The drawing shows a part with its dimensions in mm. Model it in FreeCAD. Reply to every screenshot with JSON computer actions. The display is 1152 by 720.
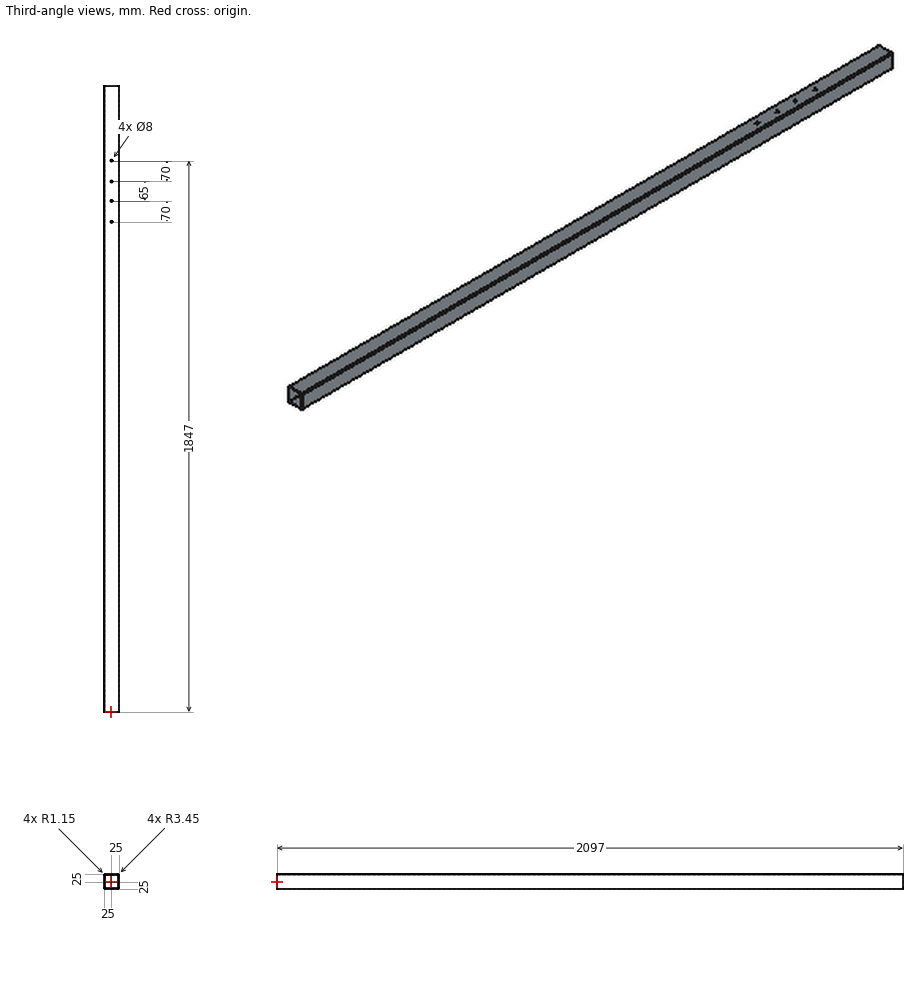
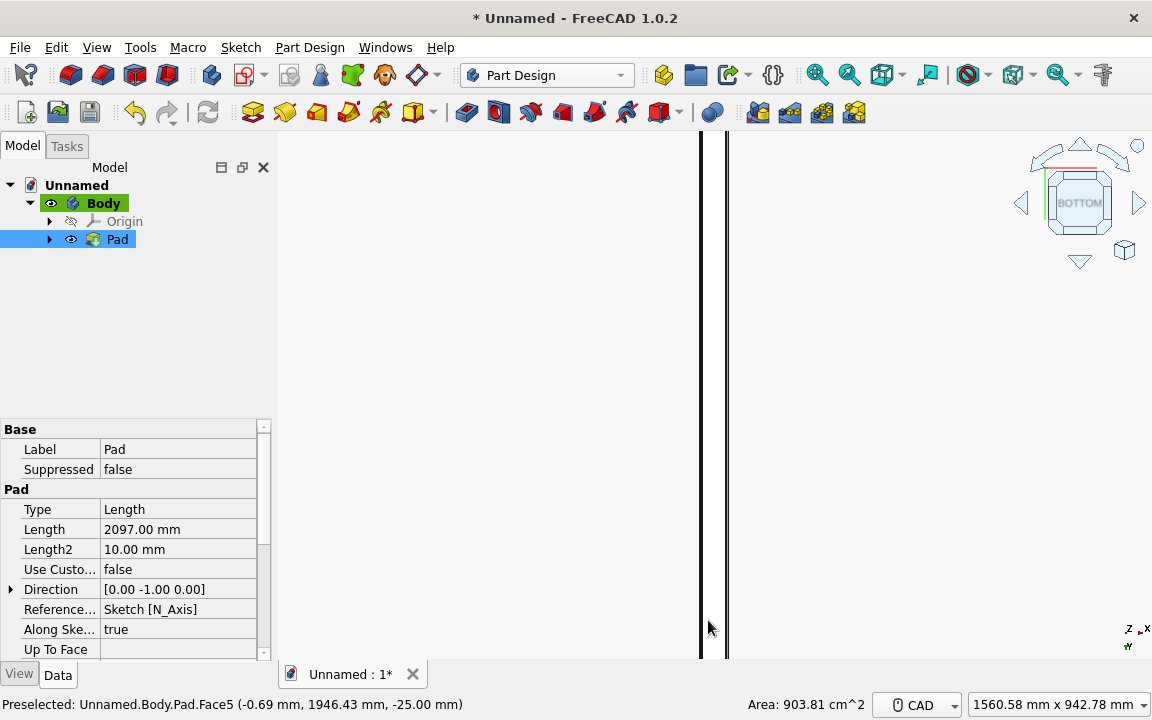
{"action": "left_click", "coordinate": [244, 76]}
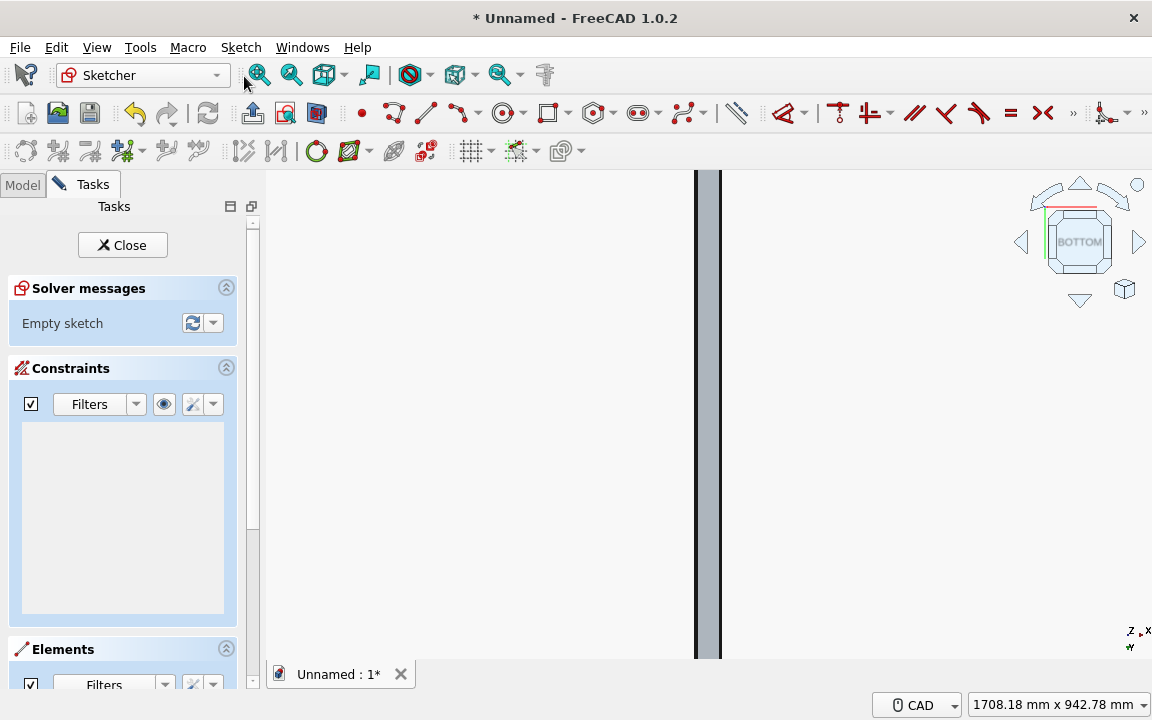
{"action": "scroll", "coordinate": [748, 580], "scroll_direction": "up", "scroll_amount": 5}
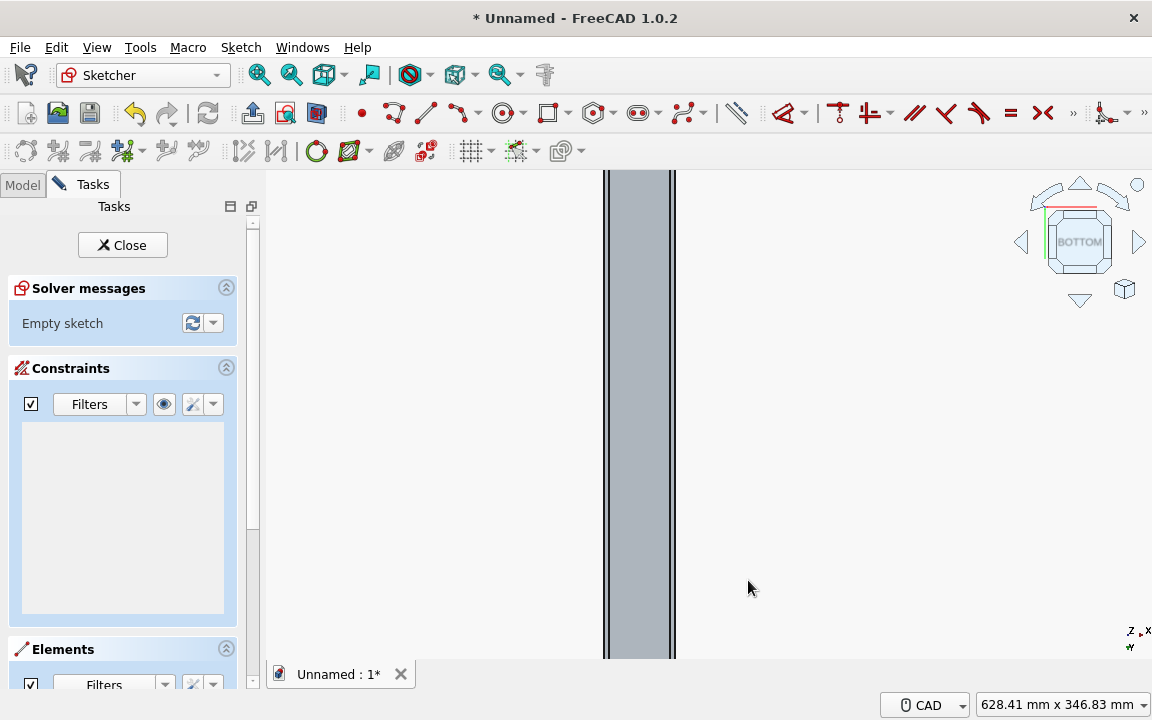
{"action": "left_click", "coordinate": [504, 114]}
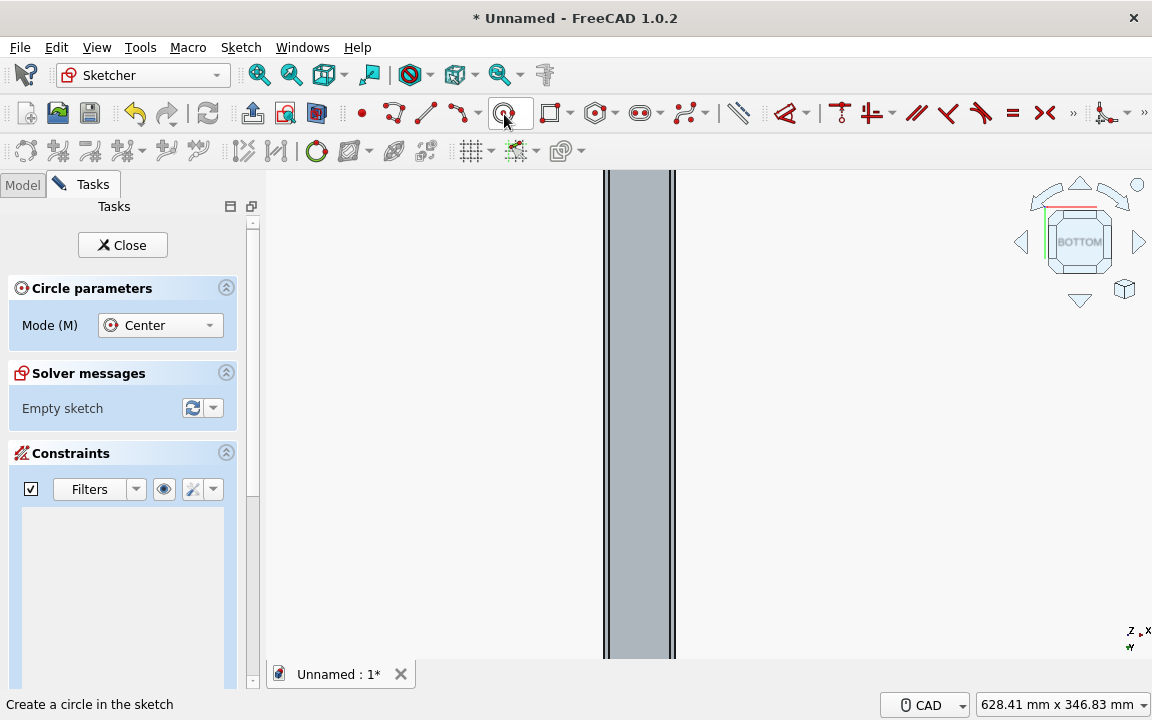
{"action": "scroll", "coordinate": [640, 557], "scroll_direction": "up", "scroll_amount": 7}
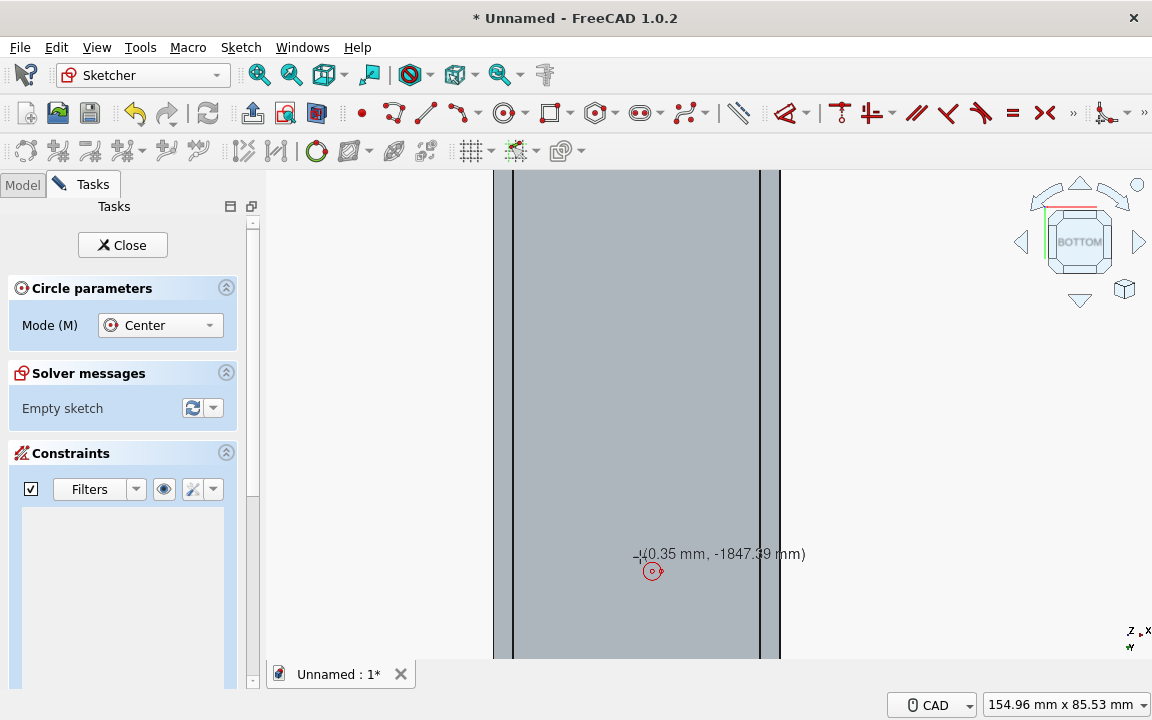
{"action": "scroll", "coordinate": [642, 560], "scroll_direction": "down", "scroll_amount": 7}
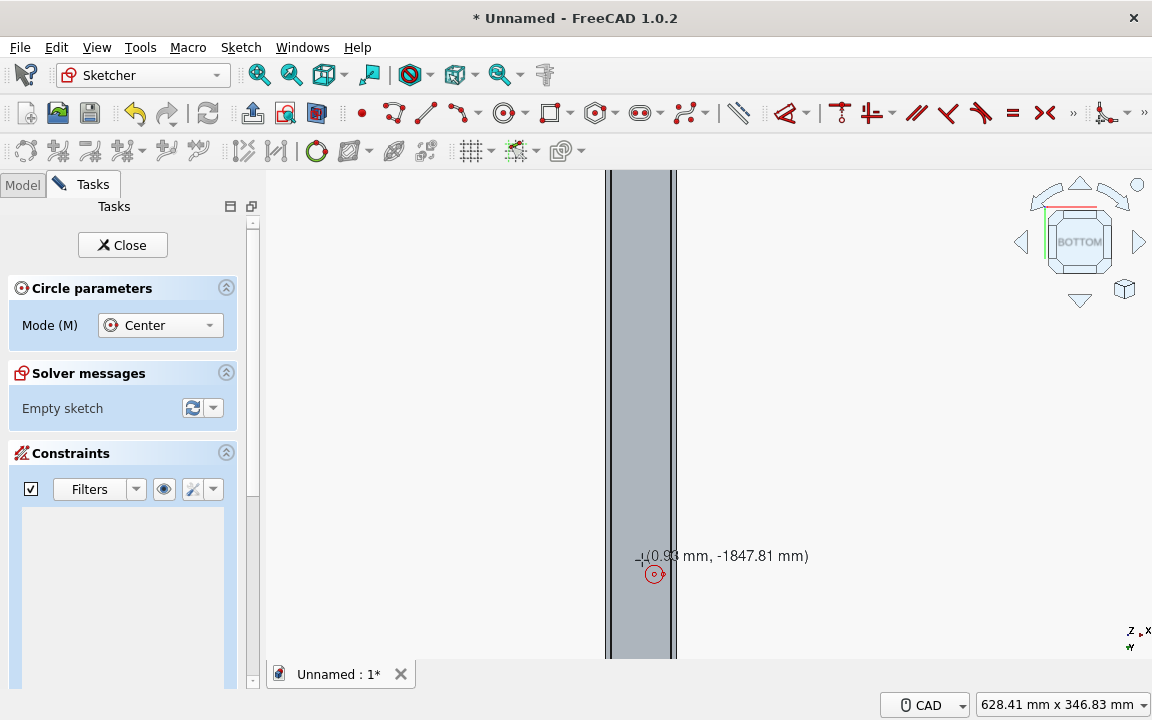
{"action": "left_click", "coordinate": [641, 560]}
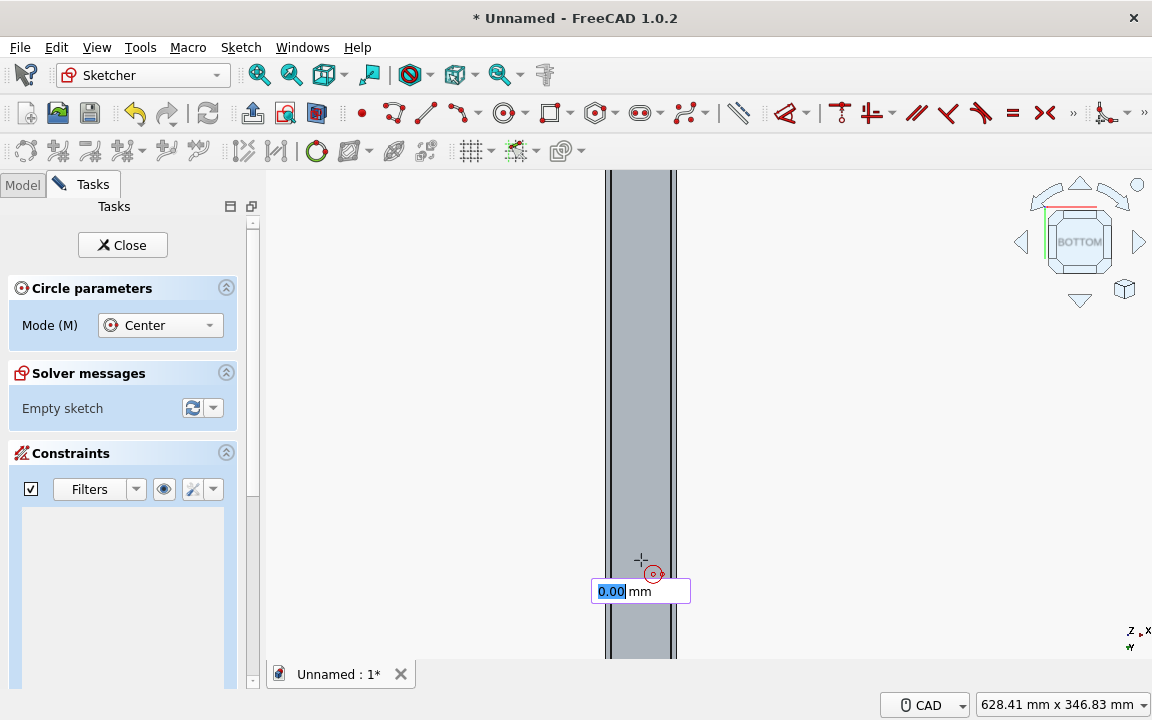
{"action": "scroll", "coordinate": [646, 558], "scroll_direction": "up", "scroll_amount": 6}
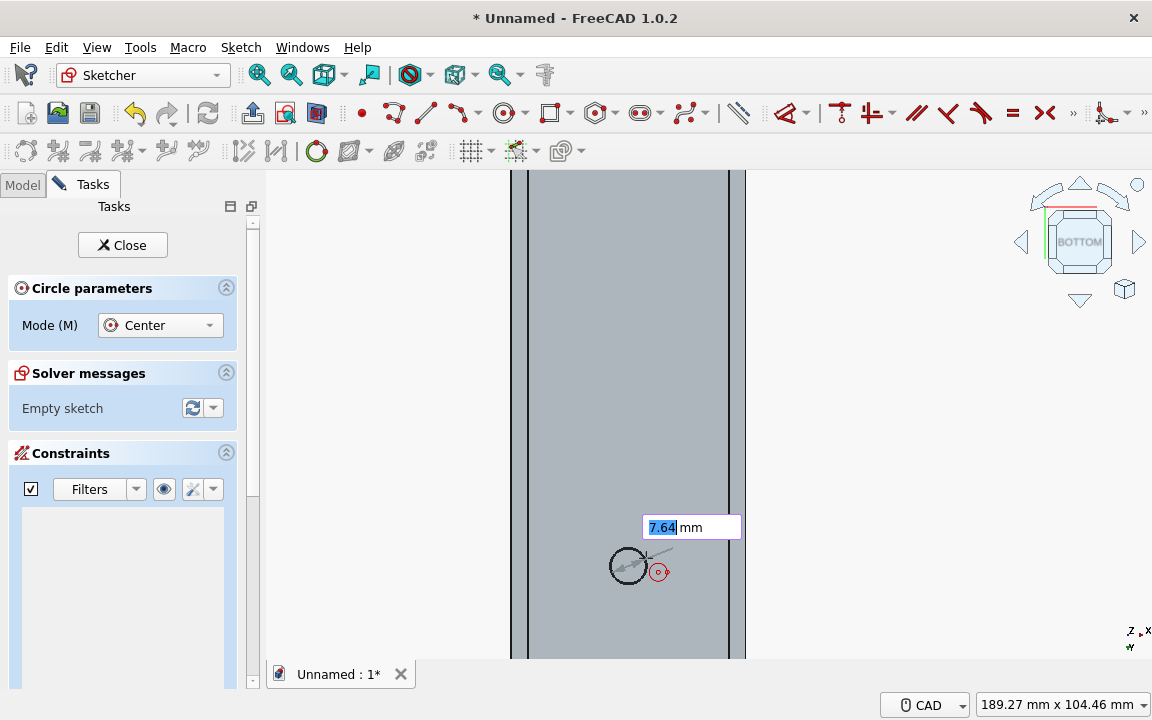
{"action": "left_click", "coordinate": [646, 555]}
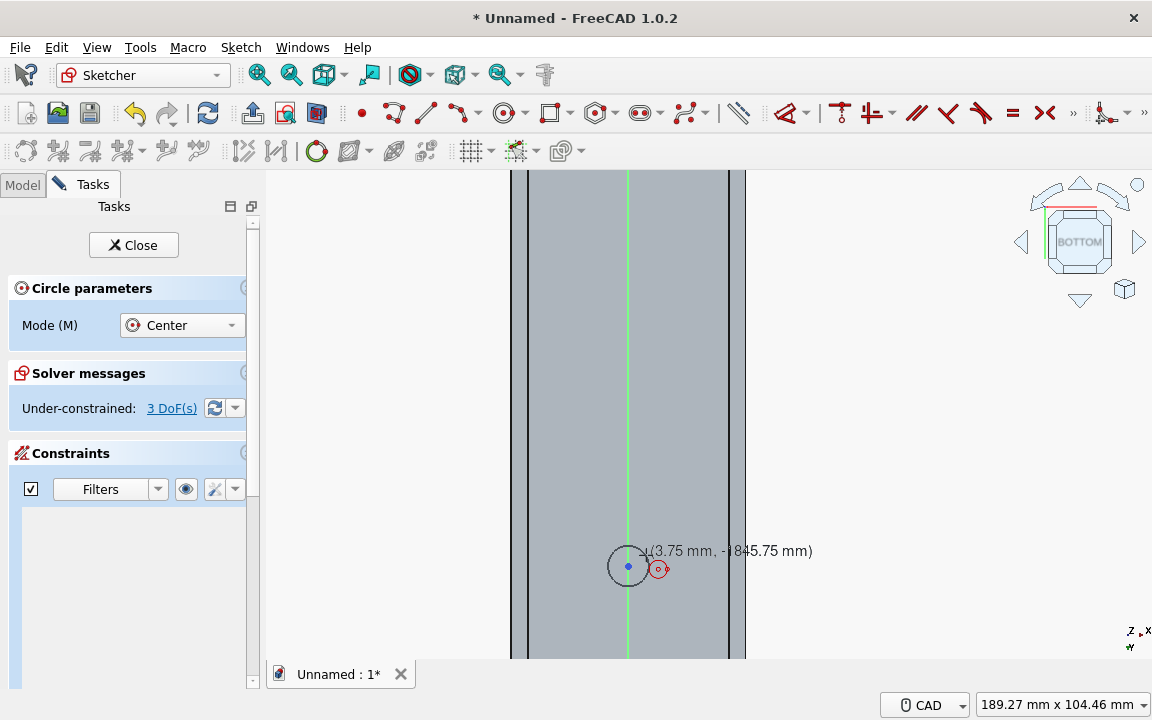
{"action": "left_click", "coordinate": [628, 234]}
{"action": "left_click", "coordinate": [646, 228]}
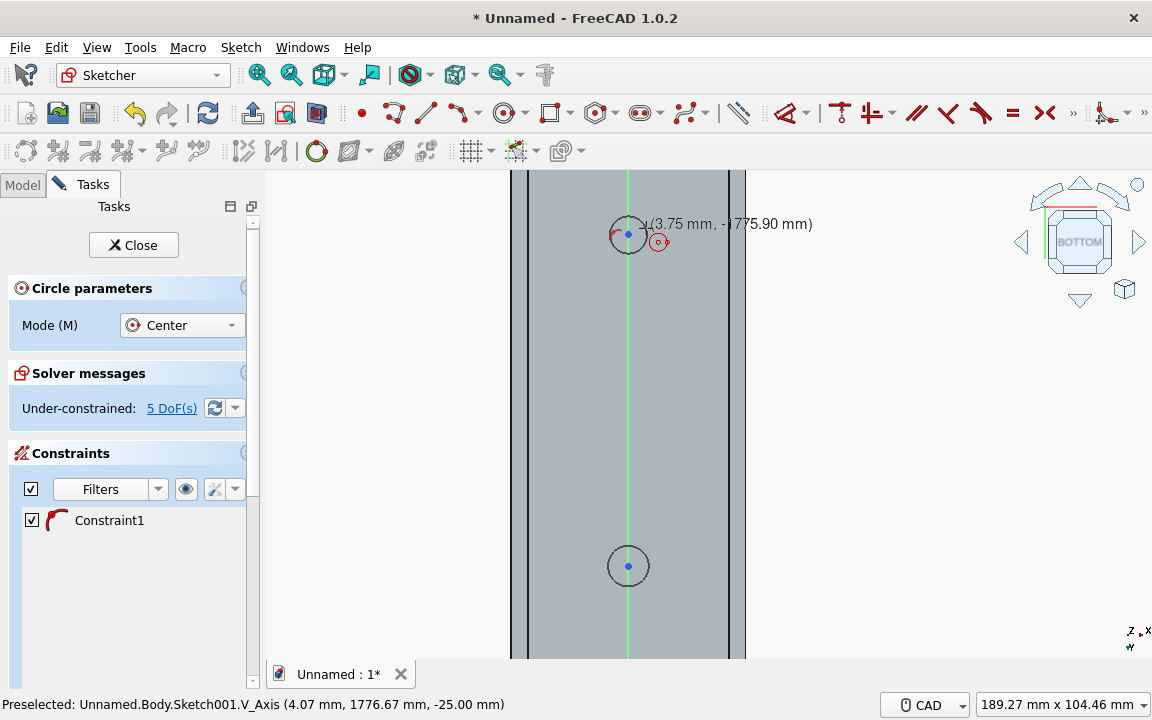
{"action": "scroll", "coordinate": [646, 558], "scroll_direction": "down", "scroll_amount": 6}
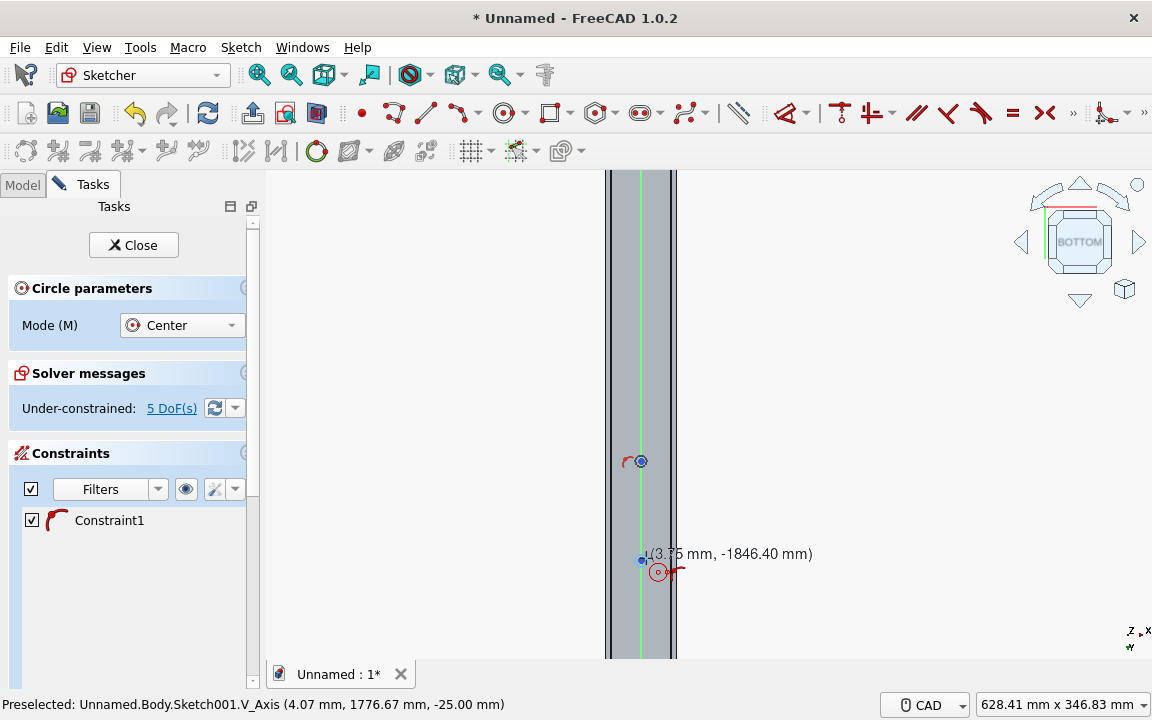
{"action": "scroll", "coordinate": [641, 369], "scroll_direction": "up", "scroll_amount": 7}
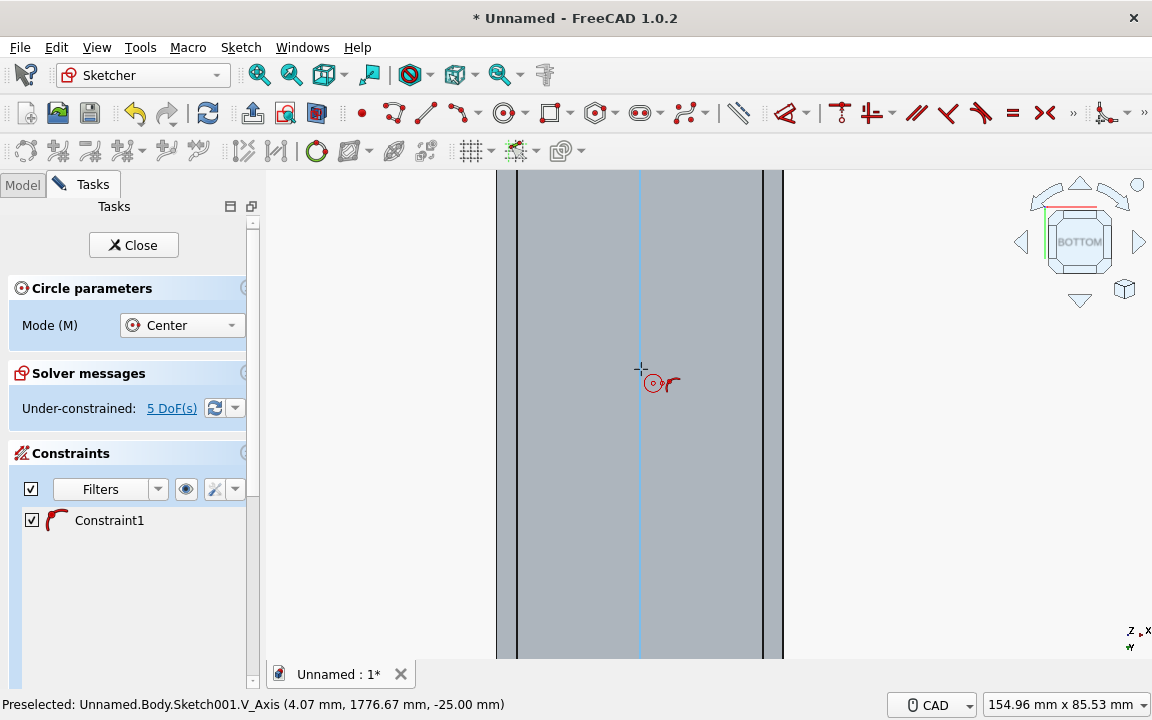
{"action": "scroll", "coordinate": [641, 368], "scroll_direction": "down", "scroll_amount": 7}